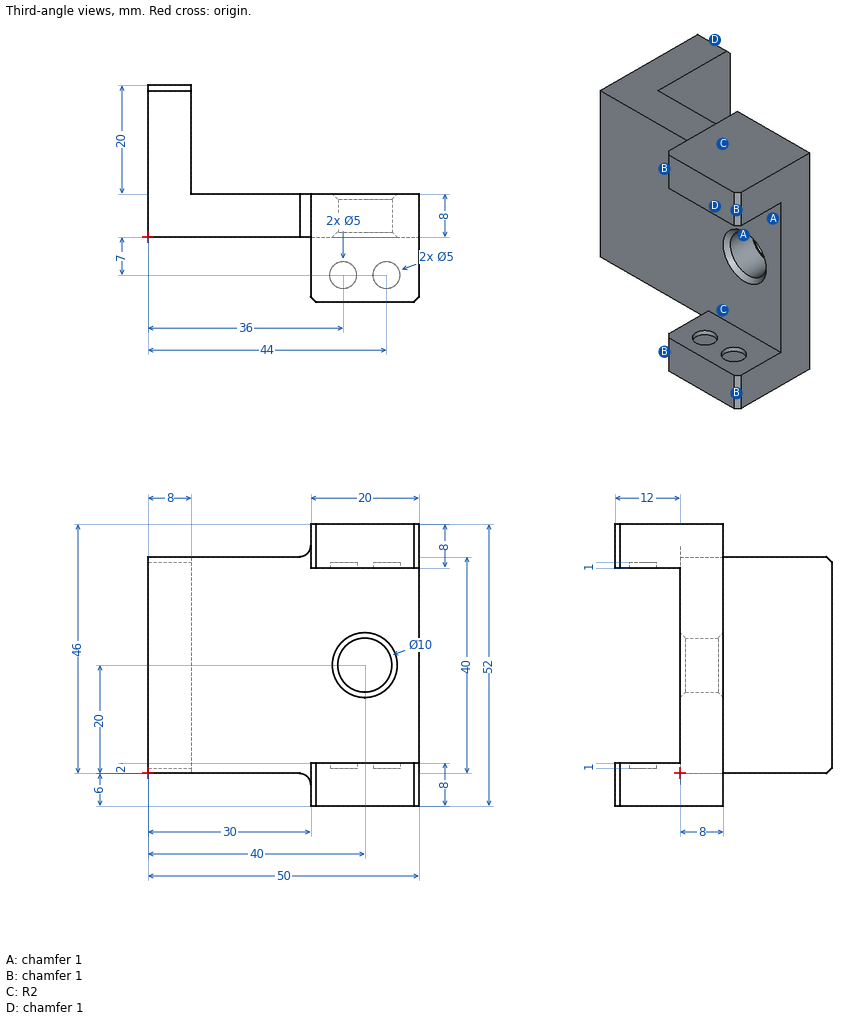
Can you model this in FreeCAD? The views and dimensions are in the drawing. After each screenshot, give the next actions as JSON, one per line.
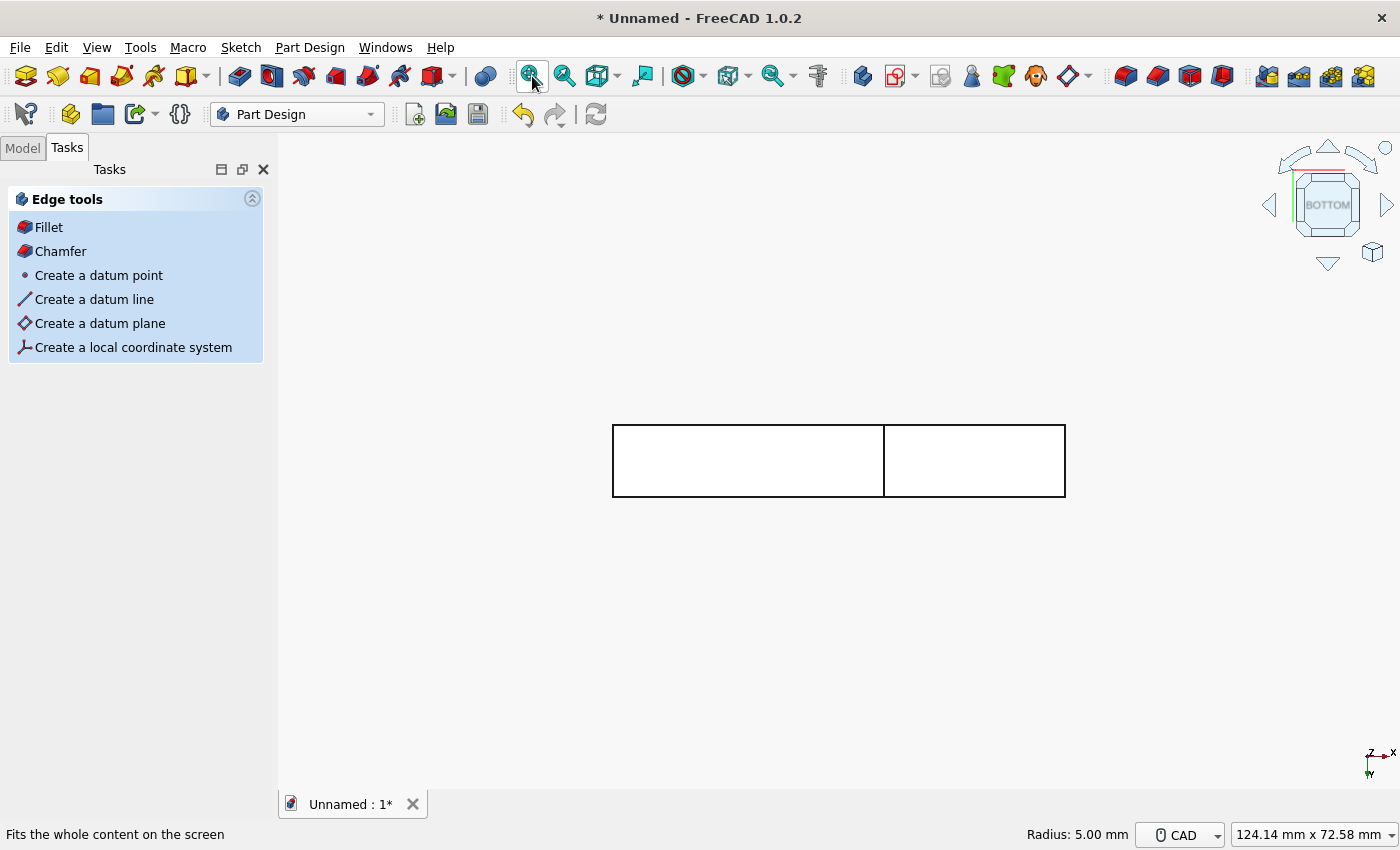
{"action": "key", "text": "4"}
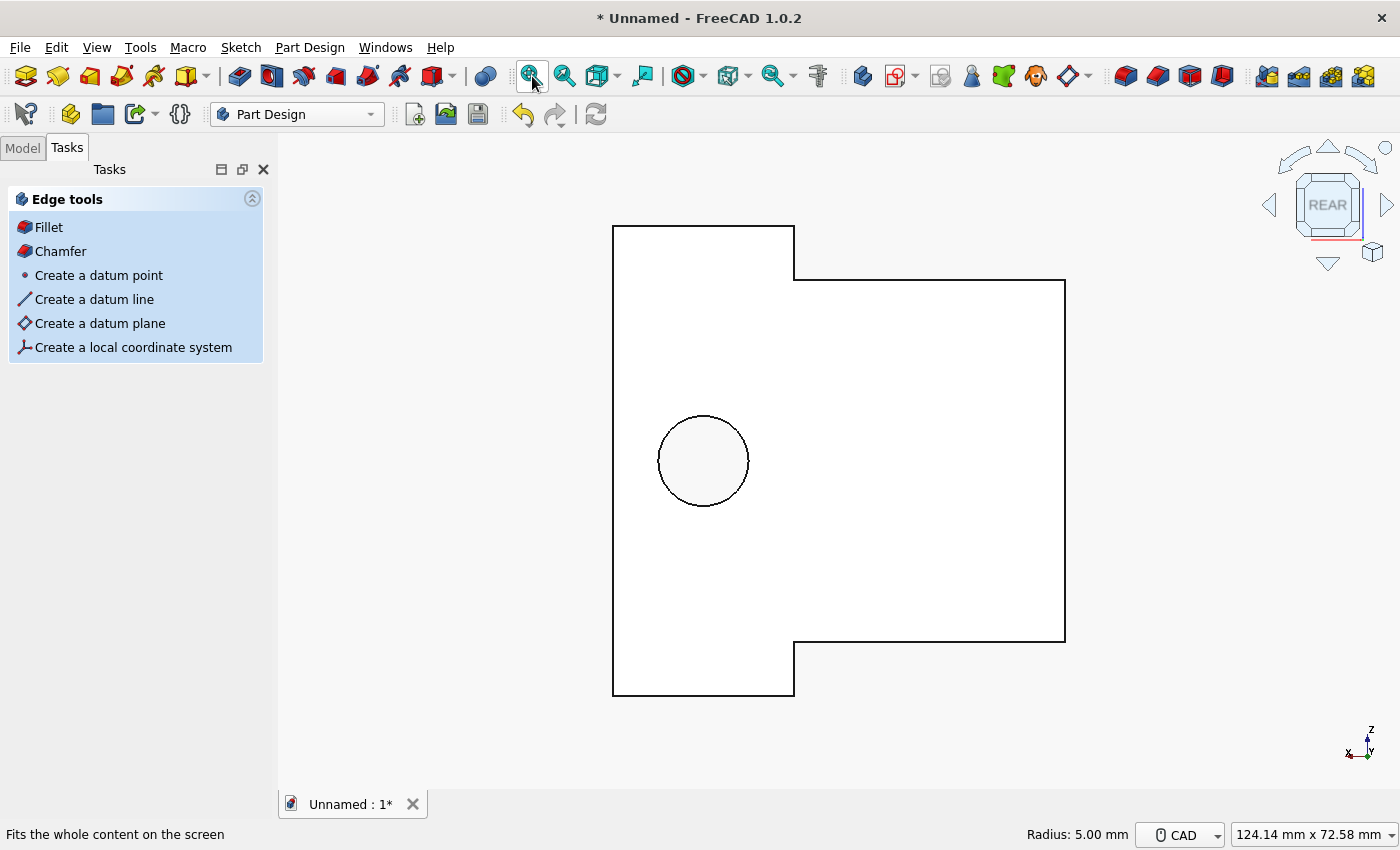
{"action": "left_click", "coordinate": [740, 433], "text": "ctrl"}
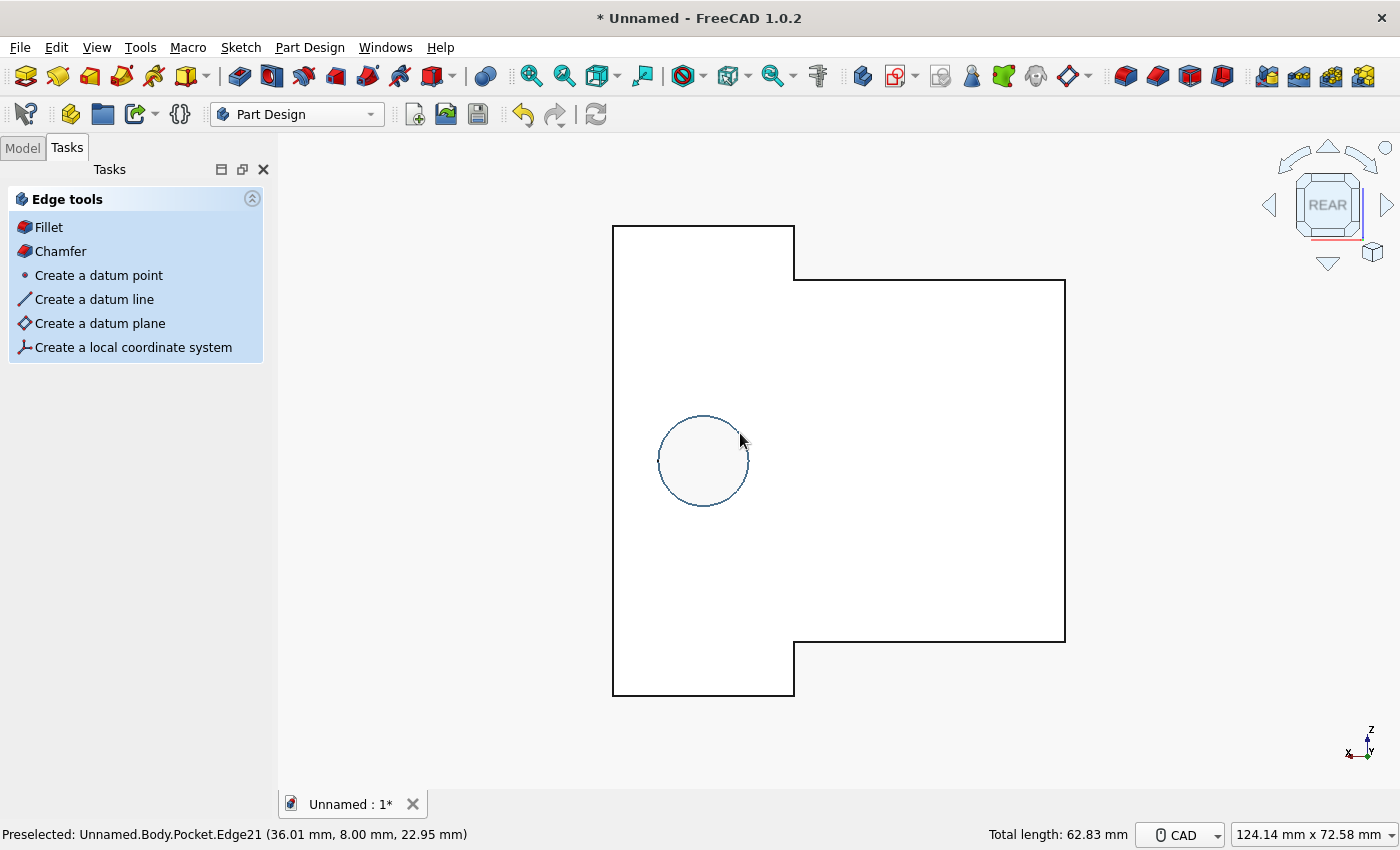
{"action": "left_click", "coordinate": [1158, 76]}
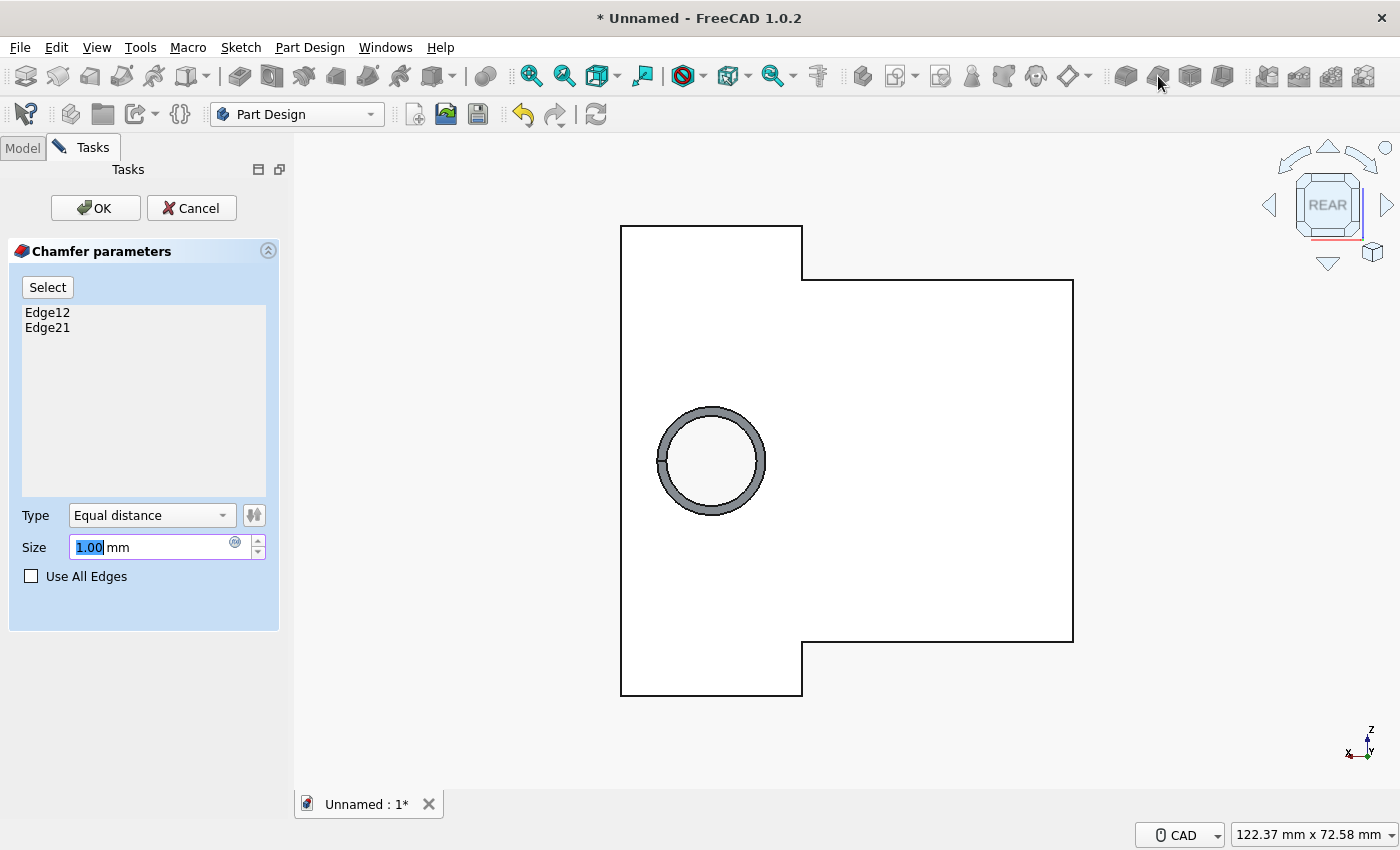
{"action": "type", "text": "1"}
{"action": "key", "text": "Tab"}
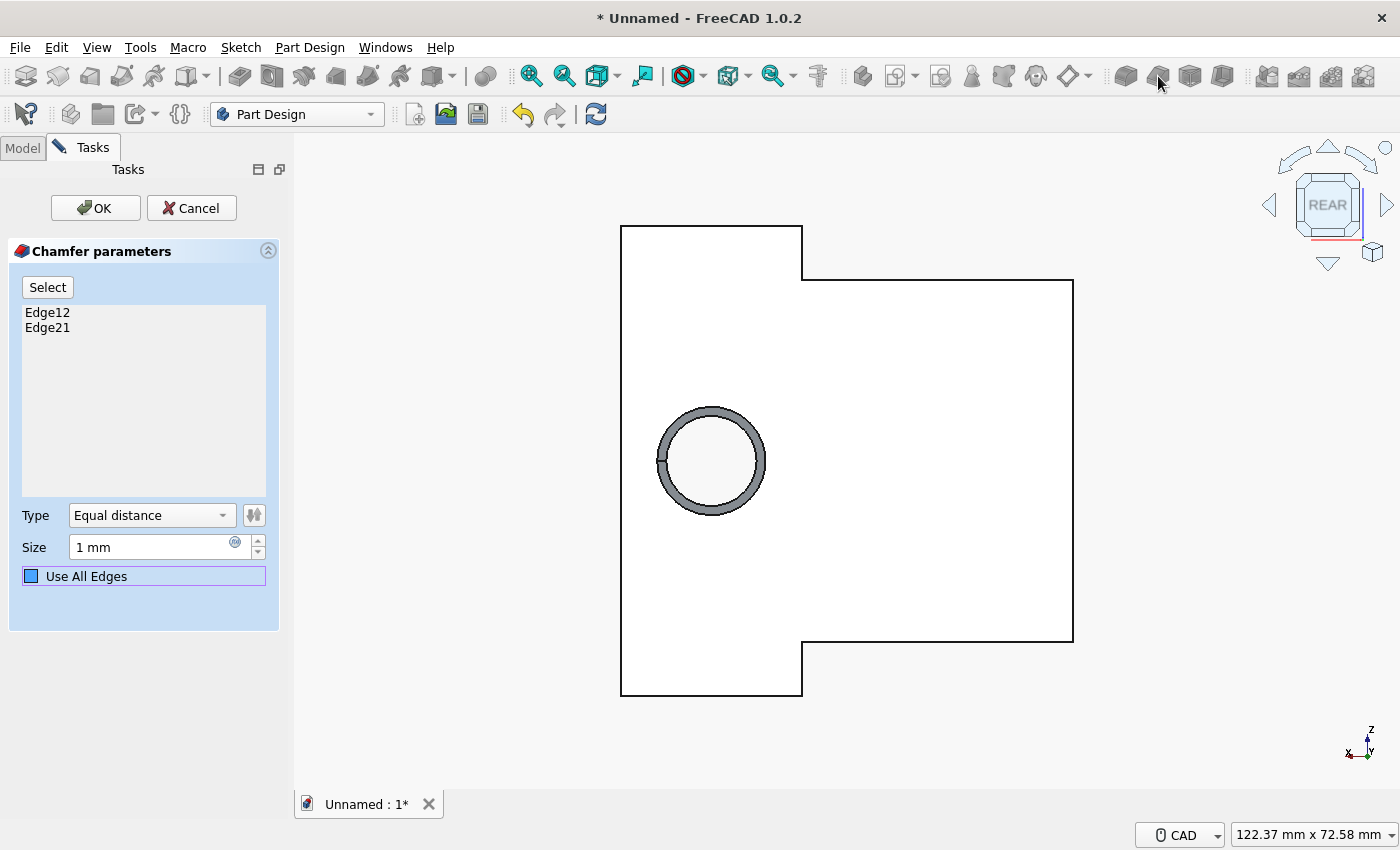
{"action": "left_click", "coordinate": [96, 208]}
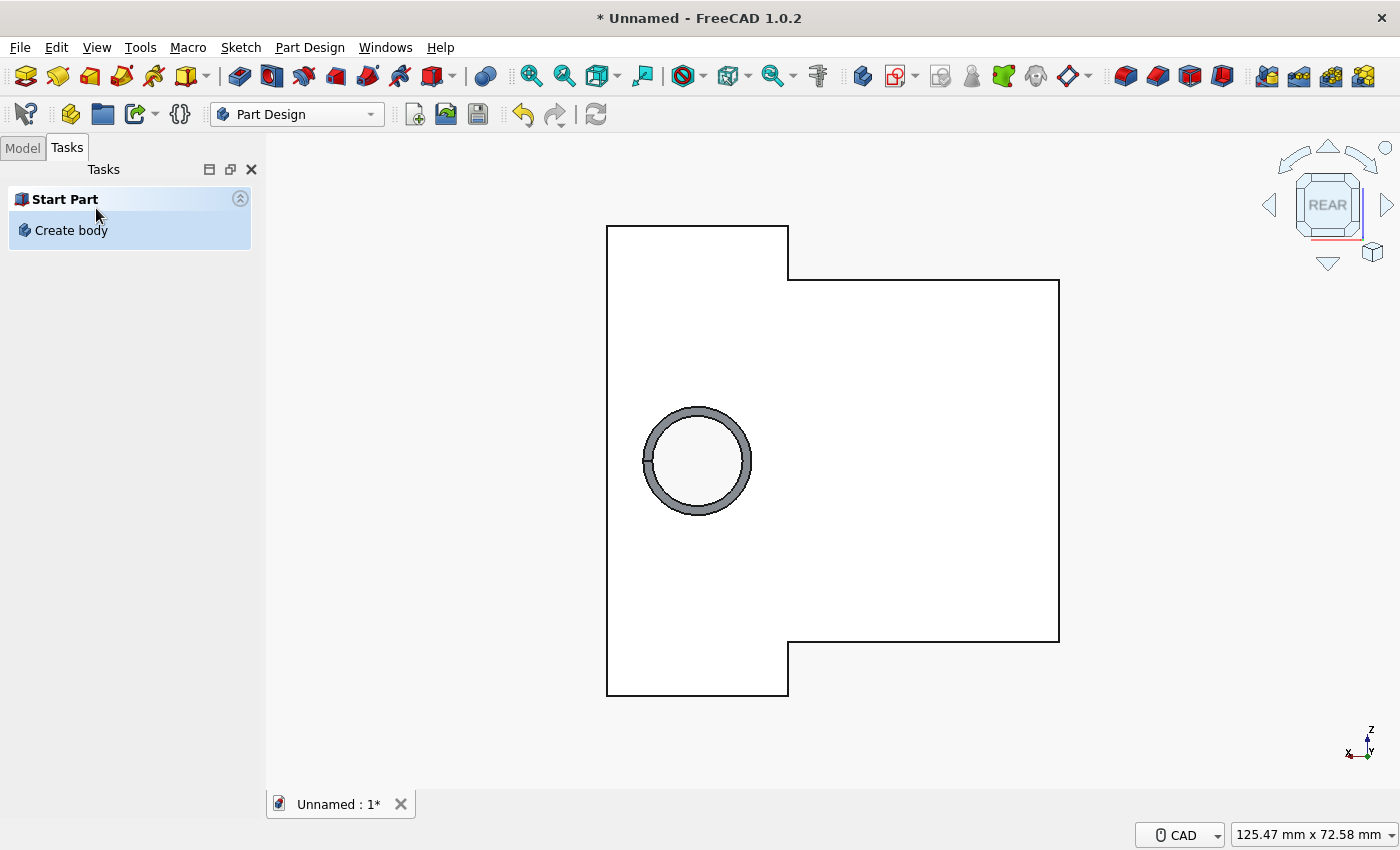
{"action": "key", "text": "0"}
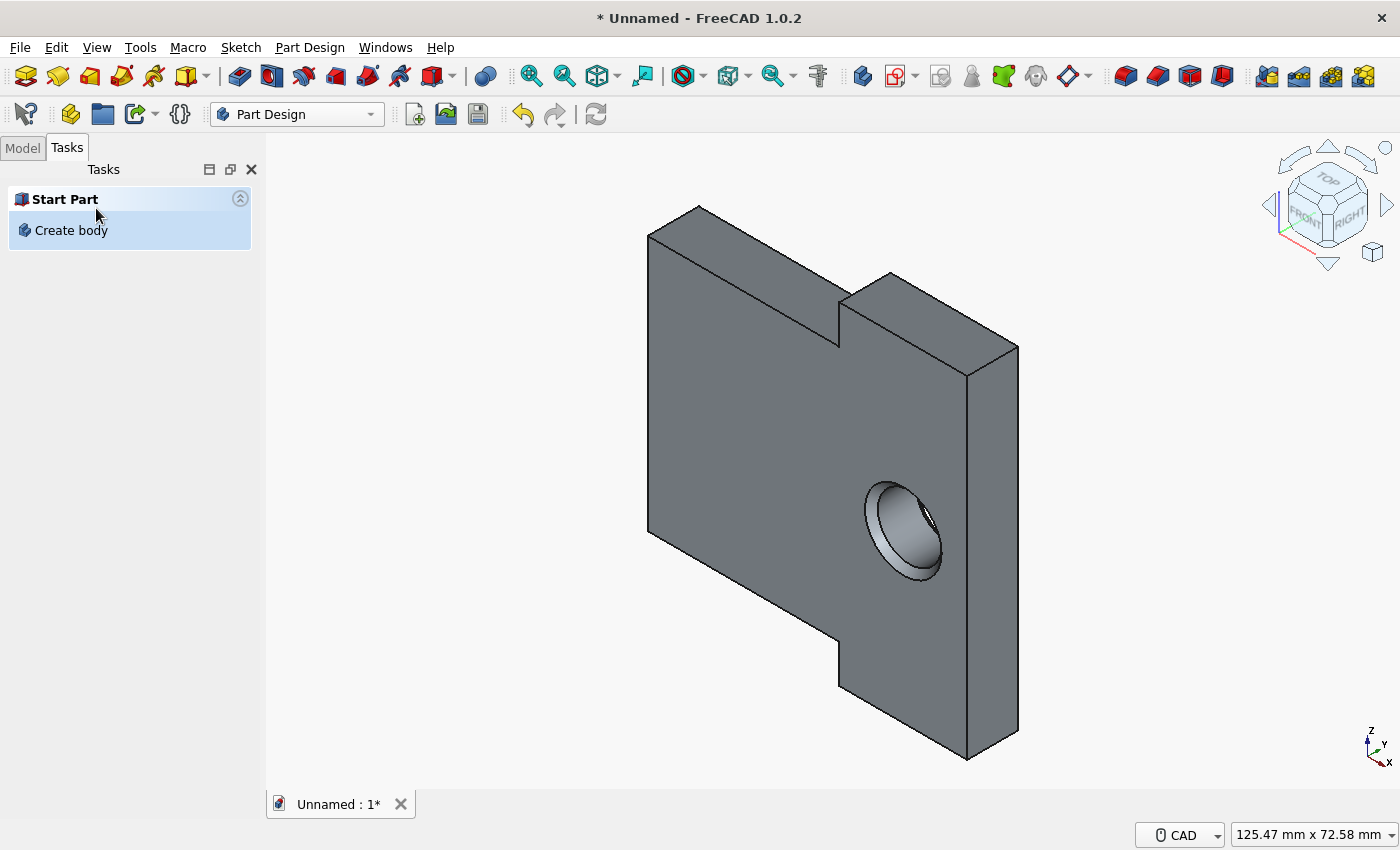
{"action": "left_click", "coordinate": [762, 448]}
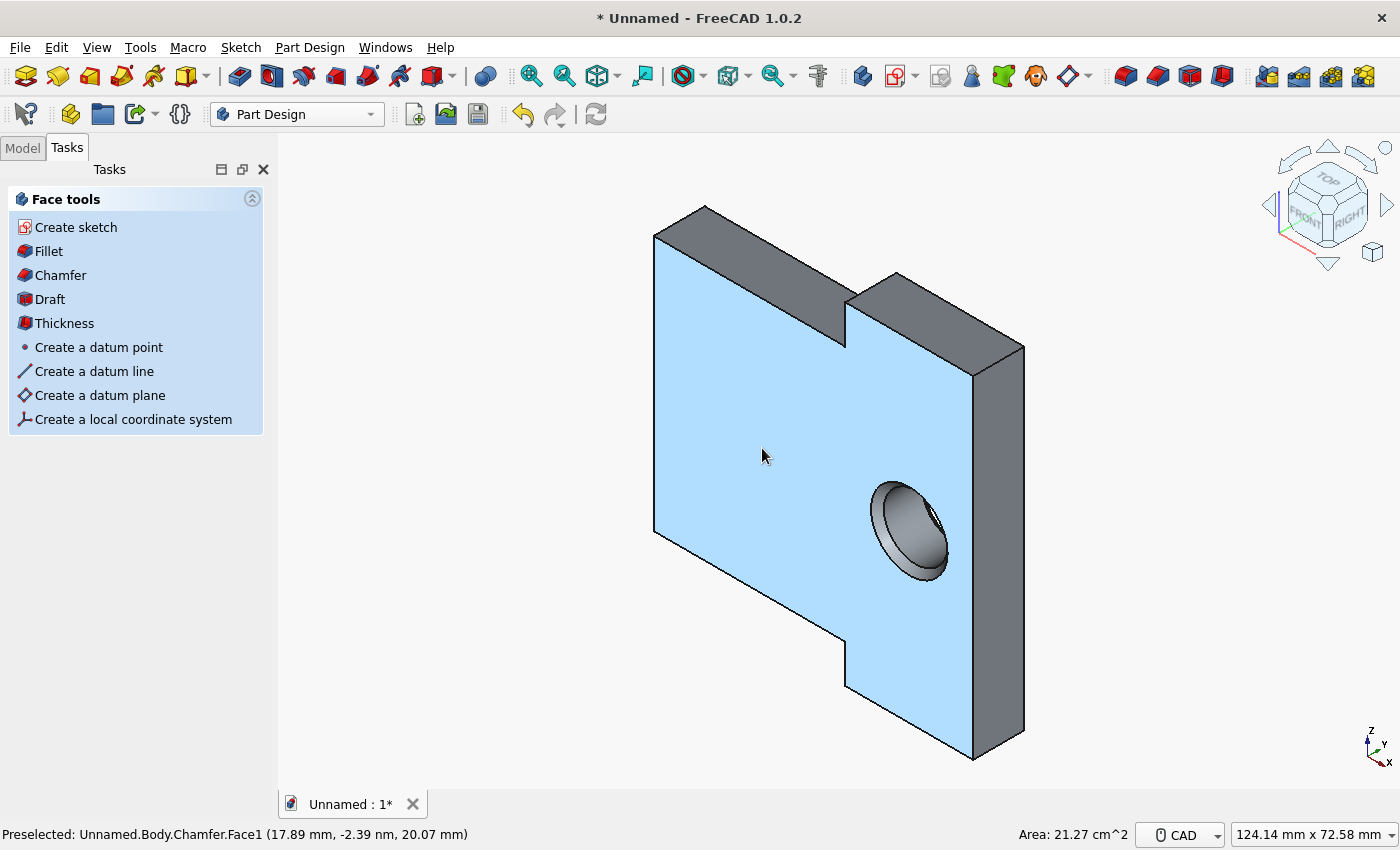
{"action": "left_click", "coordinate": [896, 76]}